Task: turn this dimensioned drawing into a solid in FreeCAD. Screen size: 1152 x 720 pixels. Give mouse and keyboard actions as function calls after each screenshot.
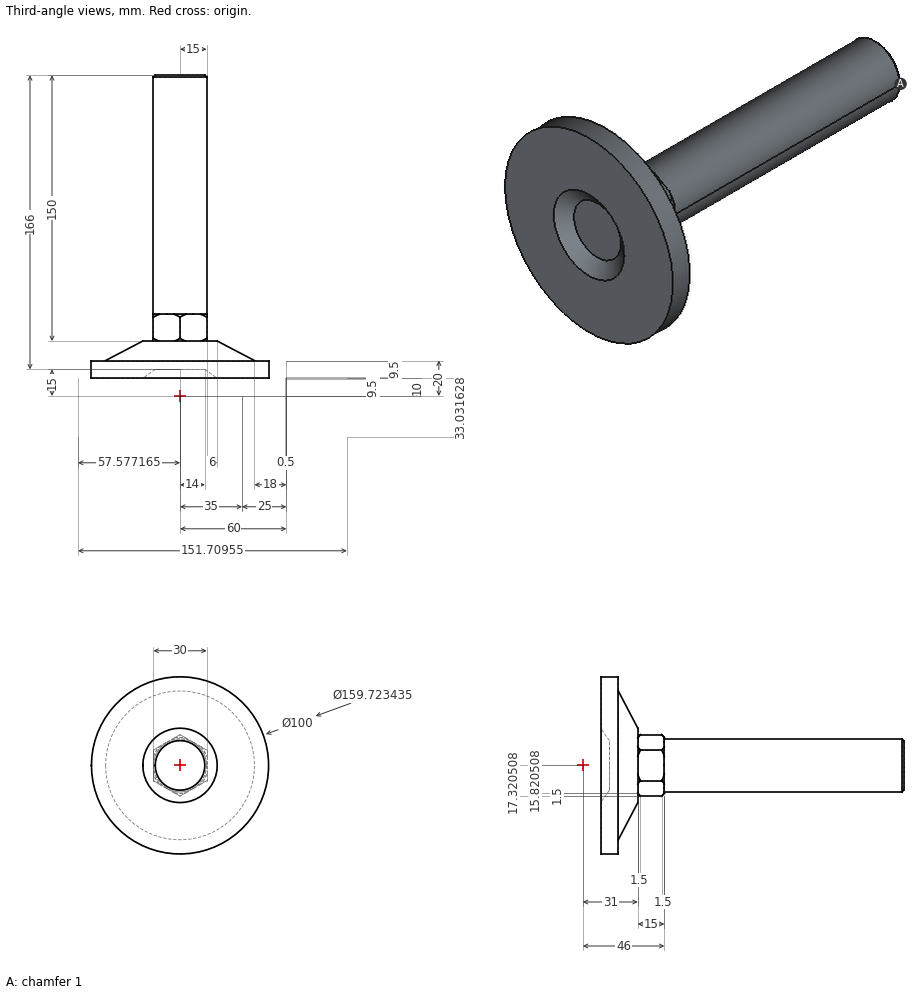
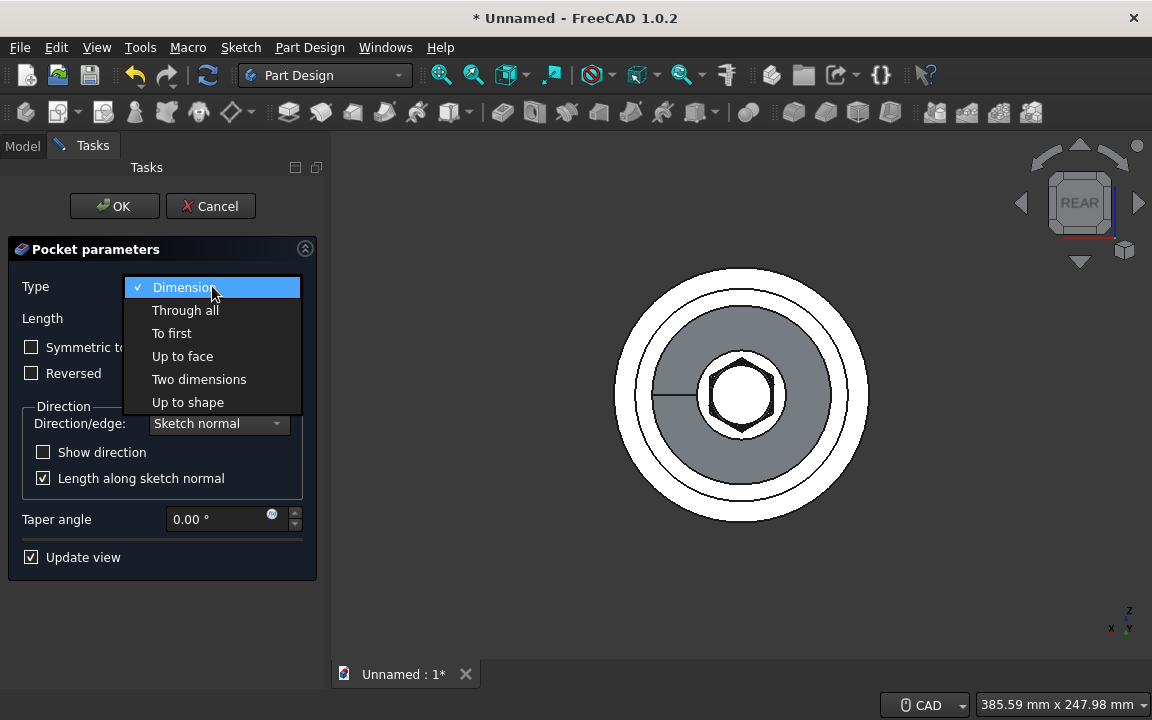
click(212, 310)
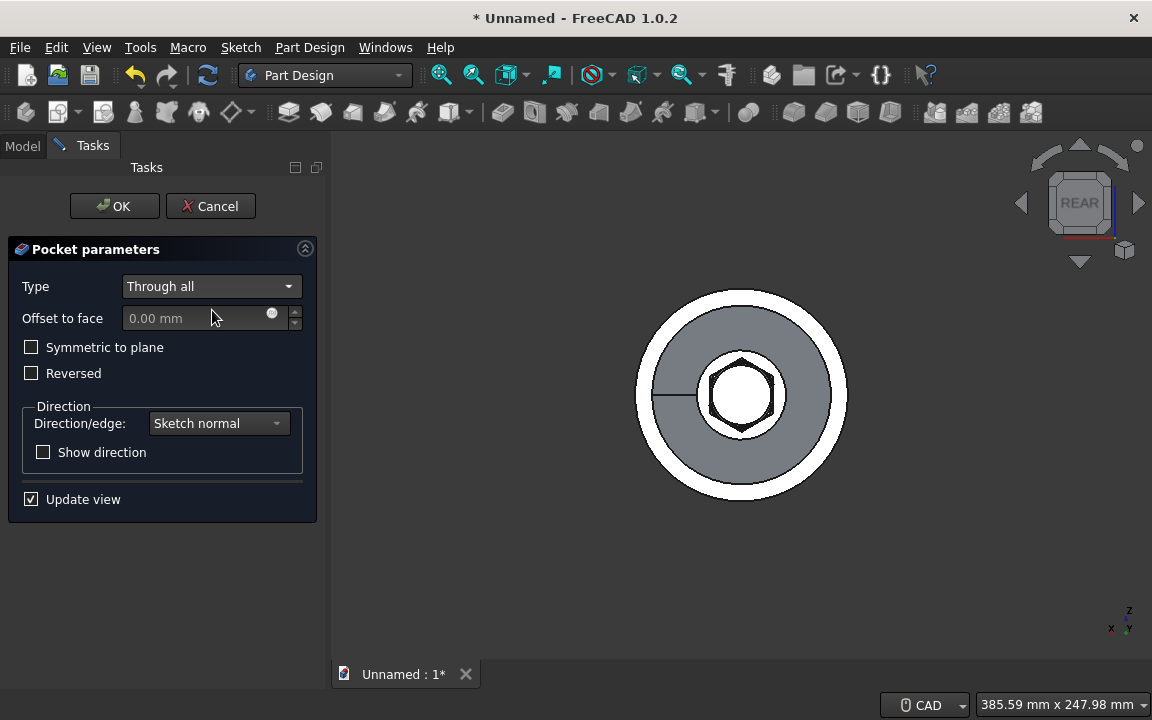
click(115, 206)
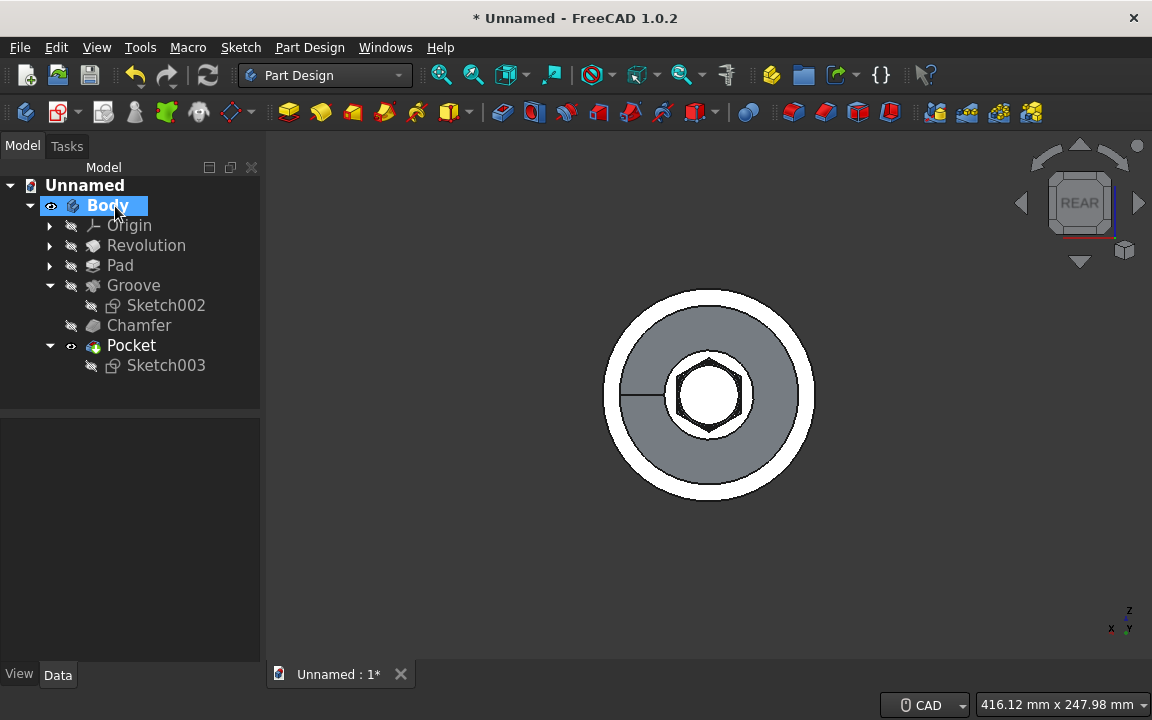
click(442, 76)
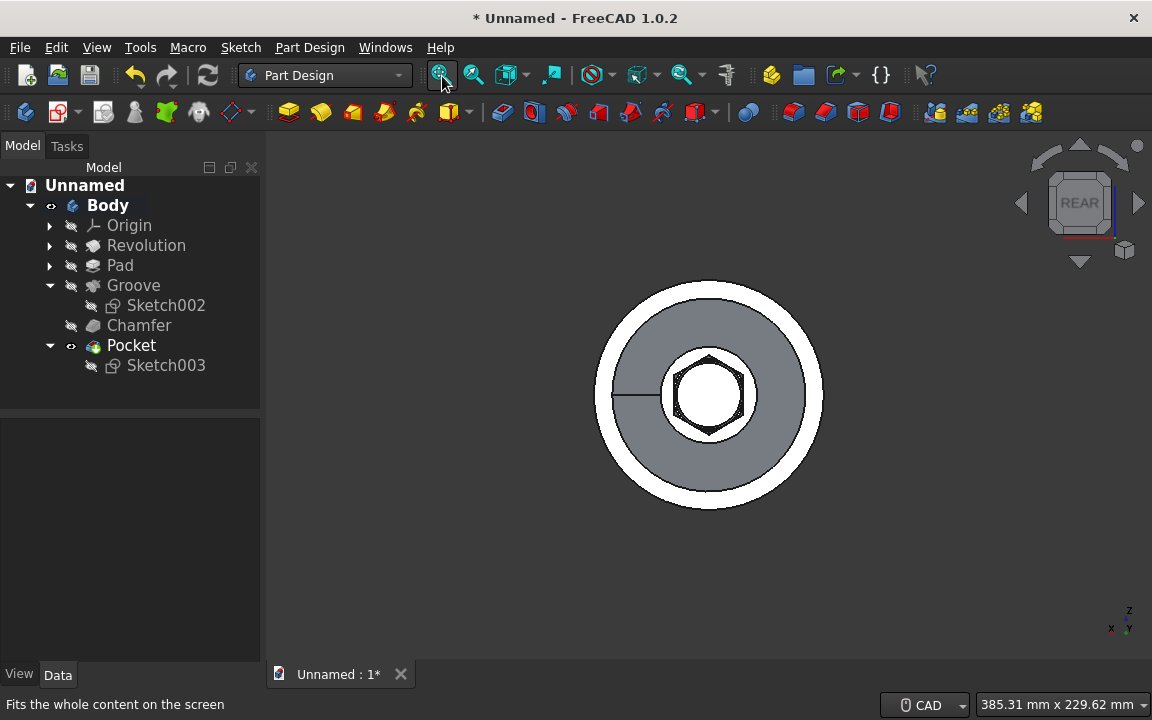
click(58, 112)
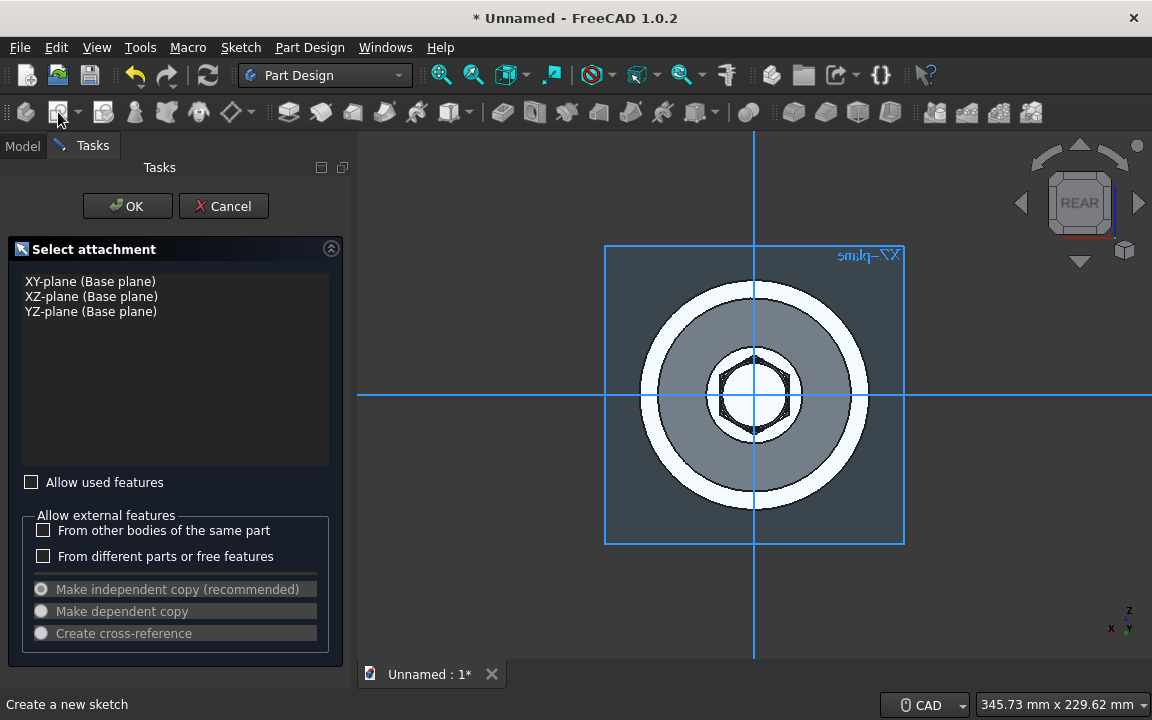
click(82, 282)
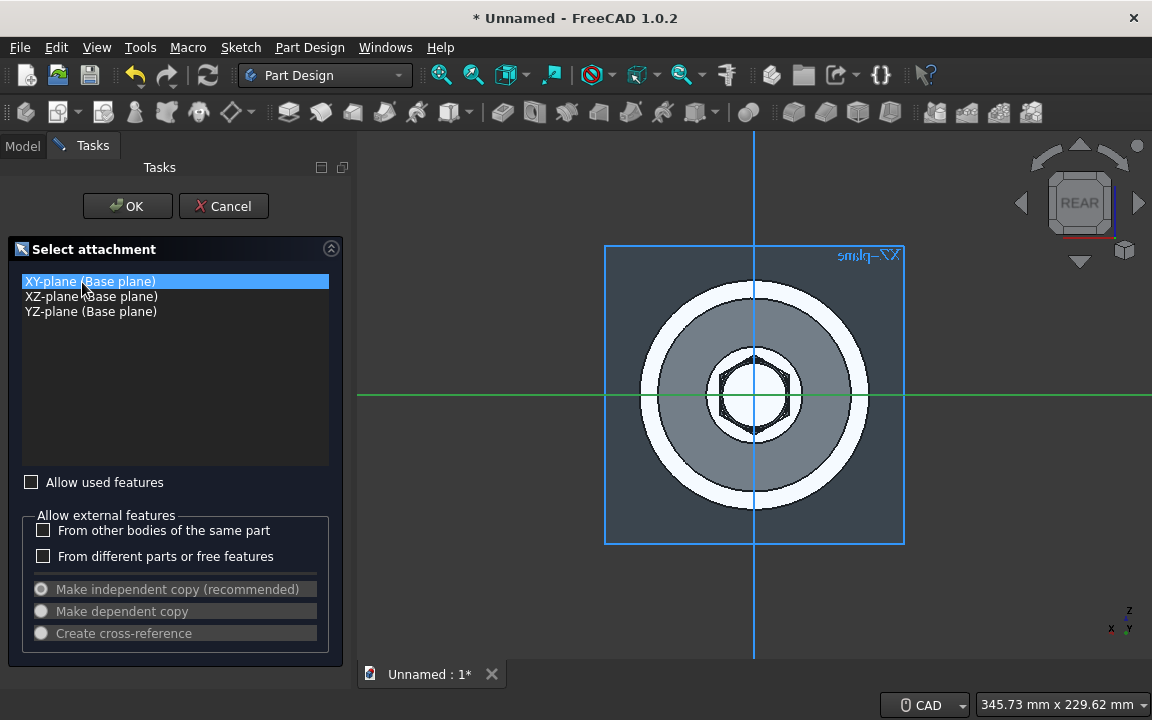
click(128, 206)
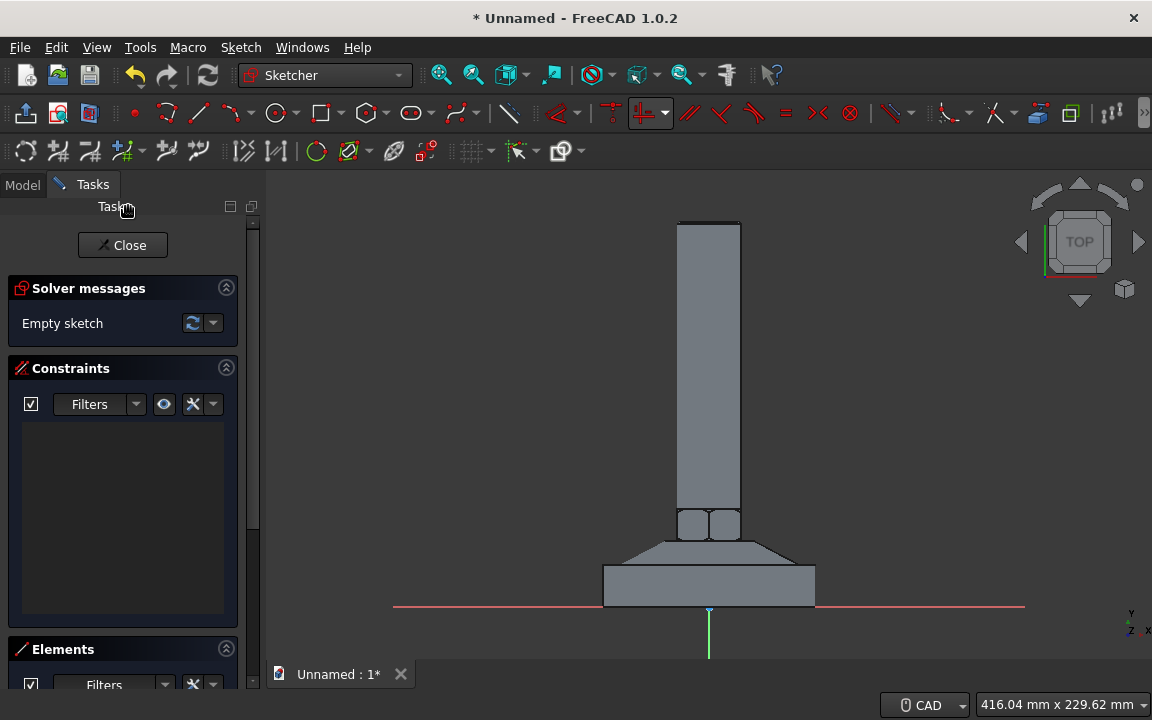
click(90, 114)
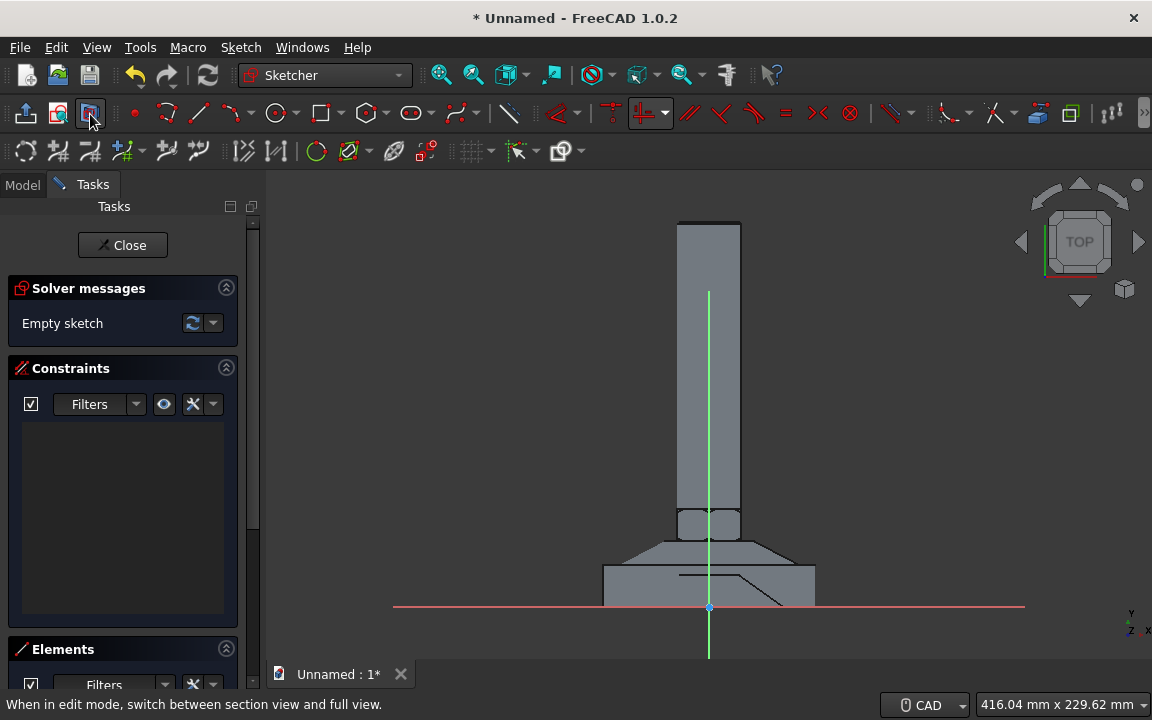
scroll(294, 198, down, 1)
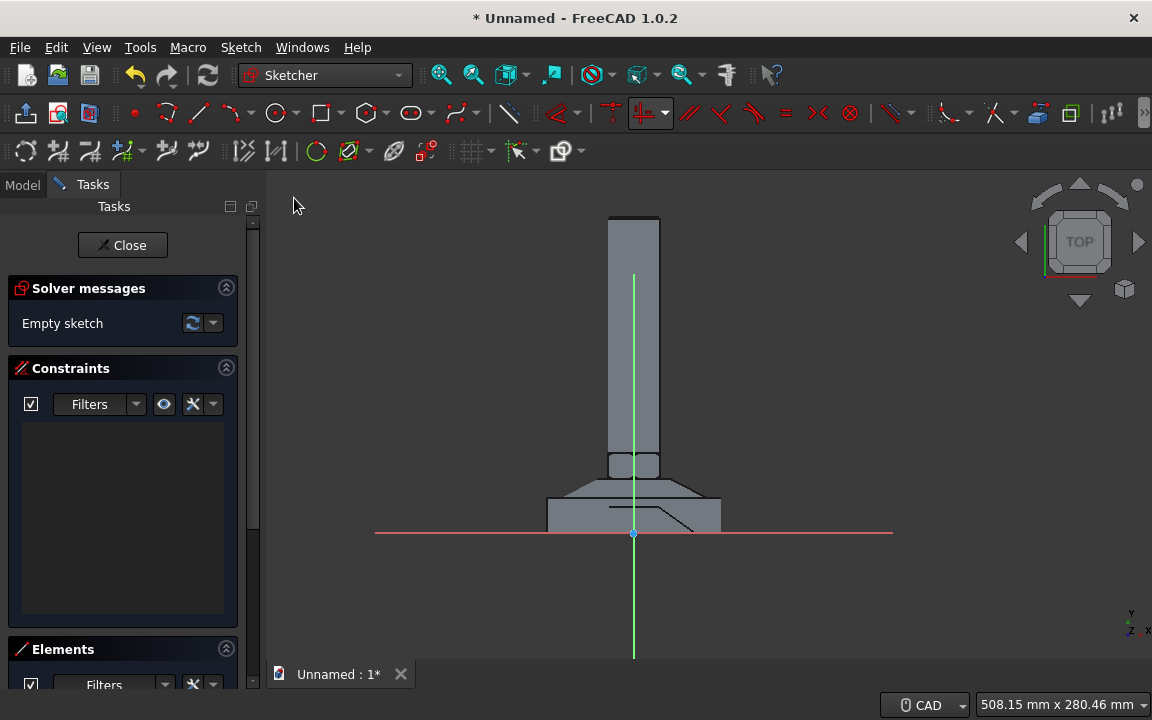
scroll(696, 631, up, 3)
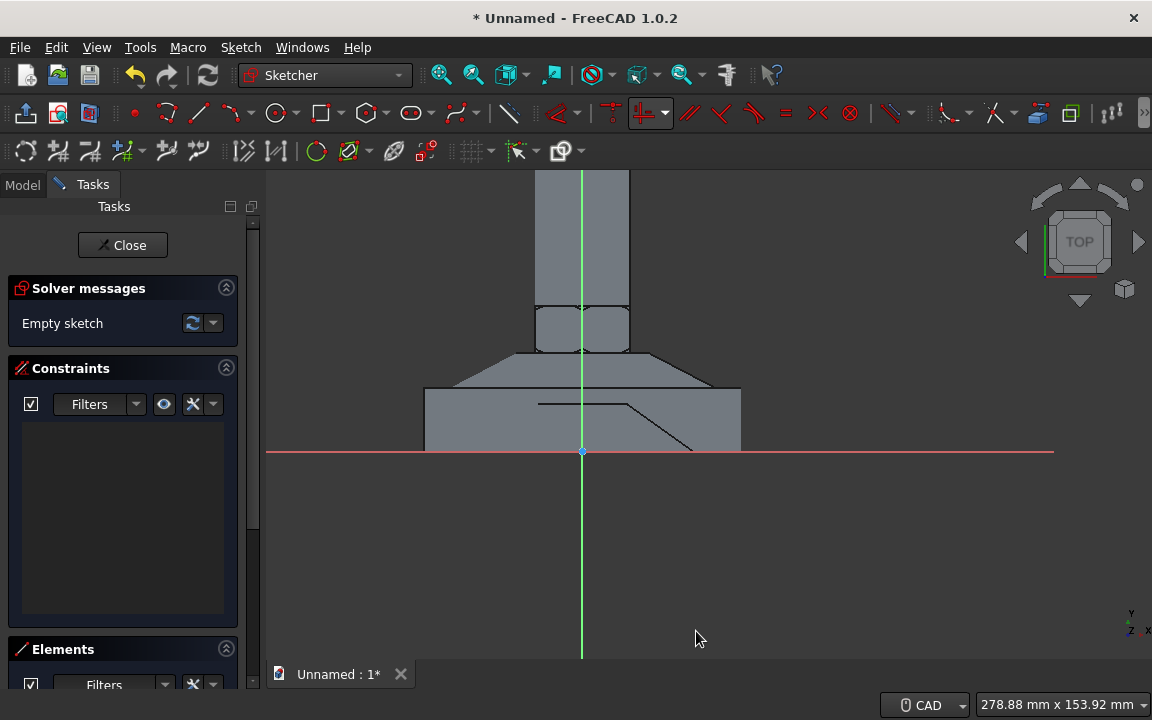
key(g)
key(r)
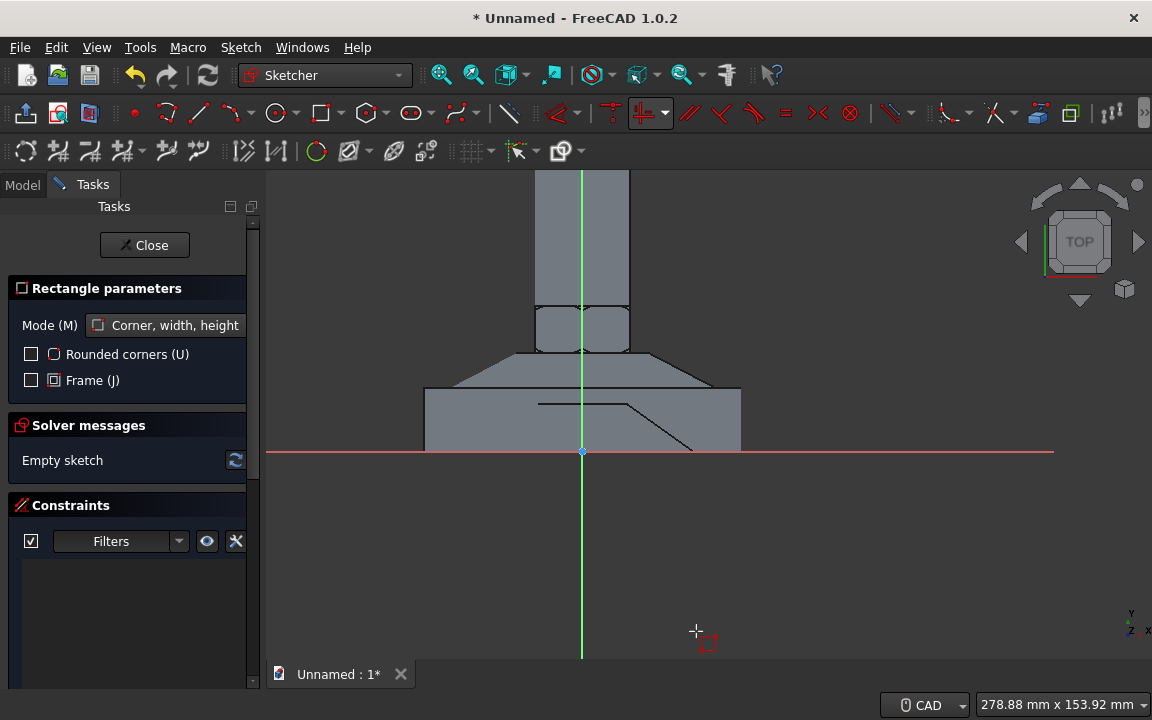
click(399, 420)
move(881, 525)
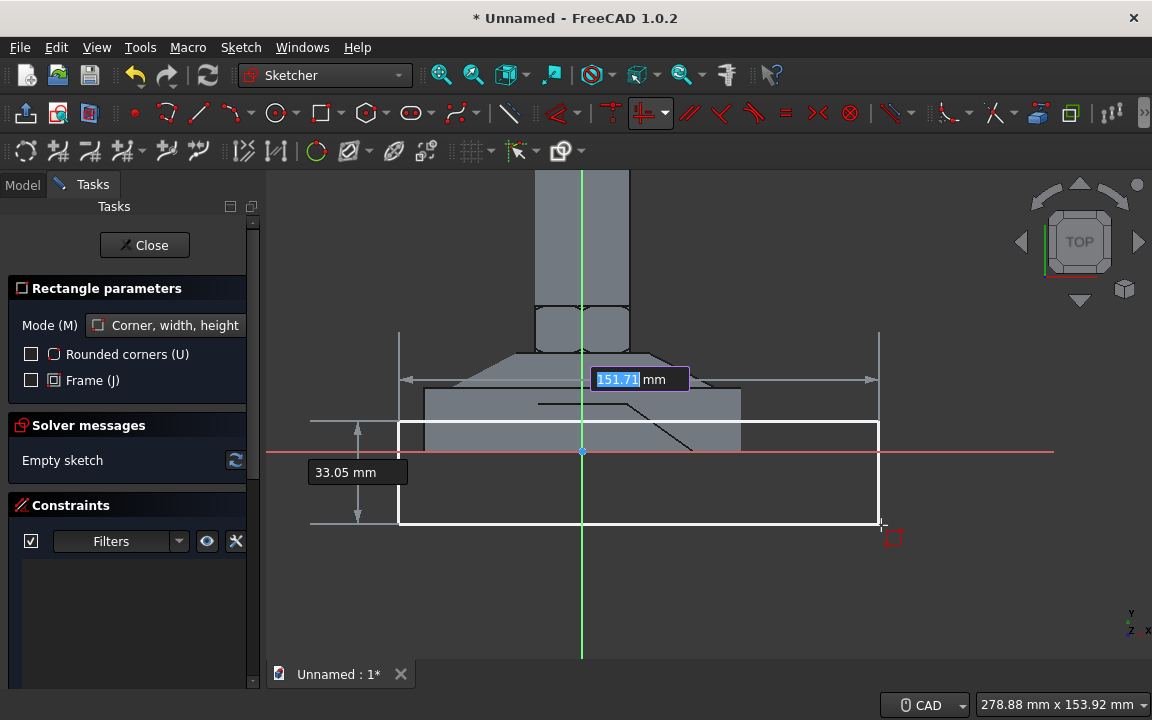
text(151.70955)
key(Tab)
text(33.031628)
key(Return)
key(Escape)